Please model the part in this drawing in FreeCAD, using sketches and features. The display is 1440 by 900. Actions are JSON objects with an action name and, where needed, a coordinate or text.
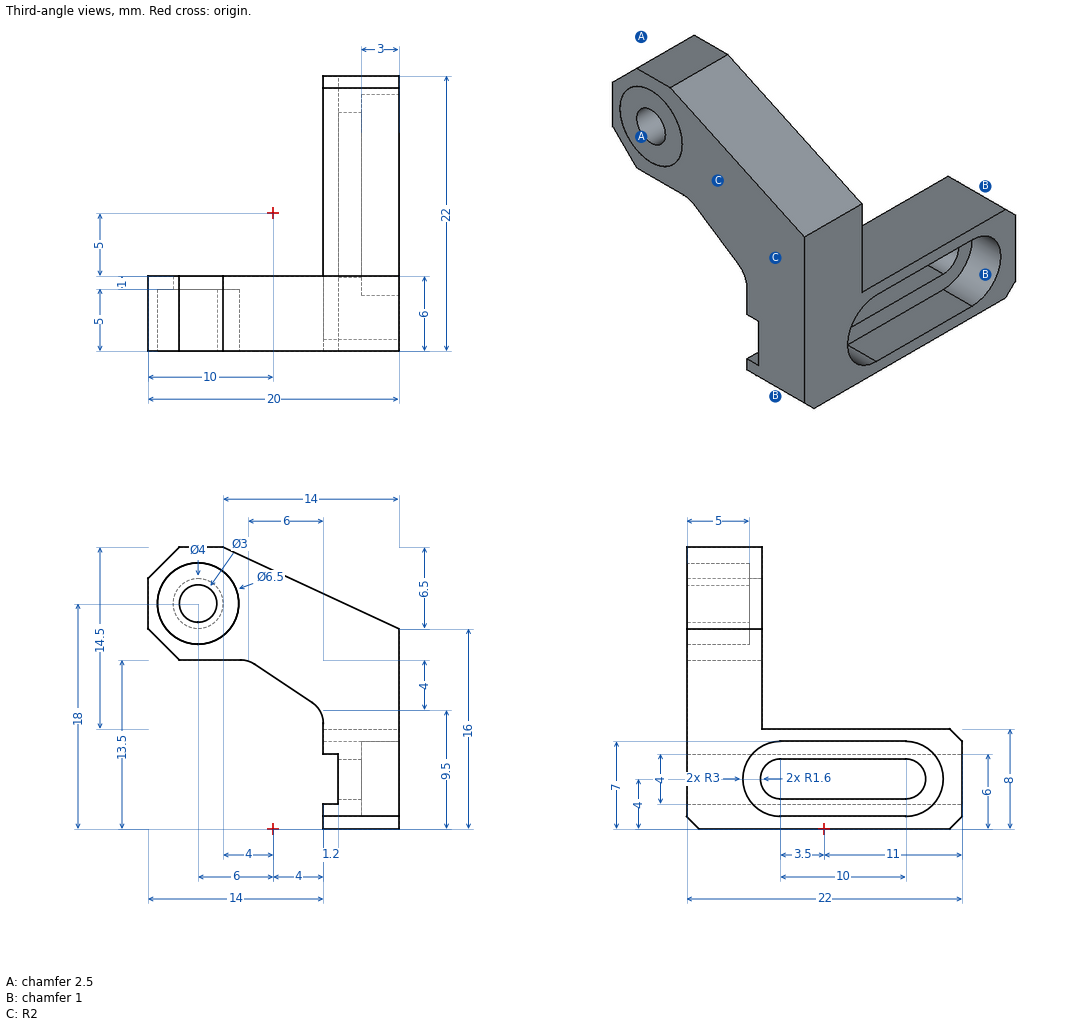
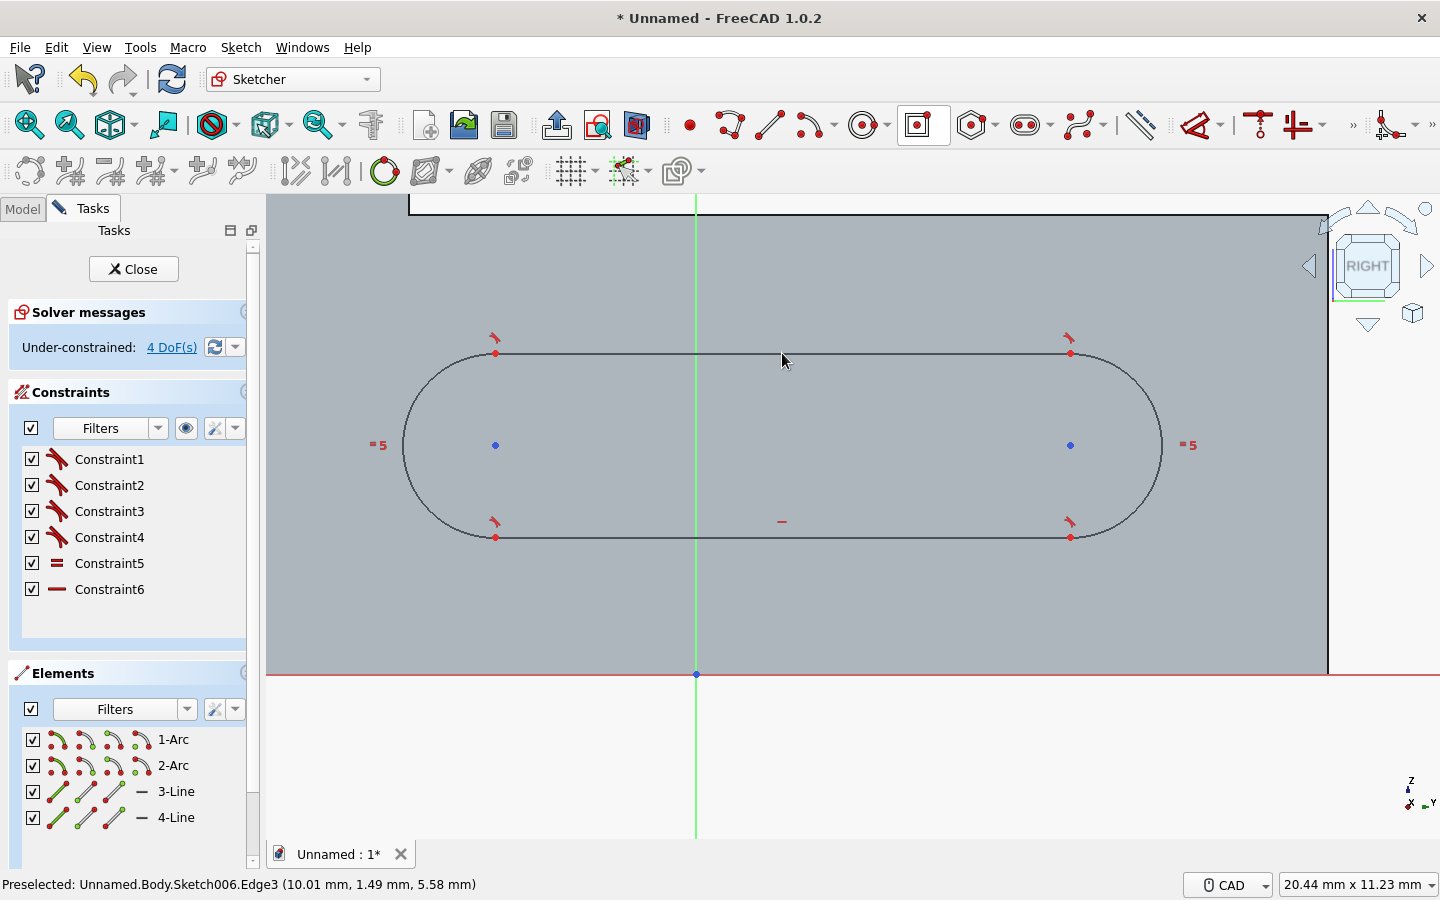
{"action": "left_click", "coordinate": [1196, 126]}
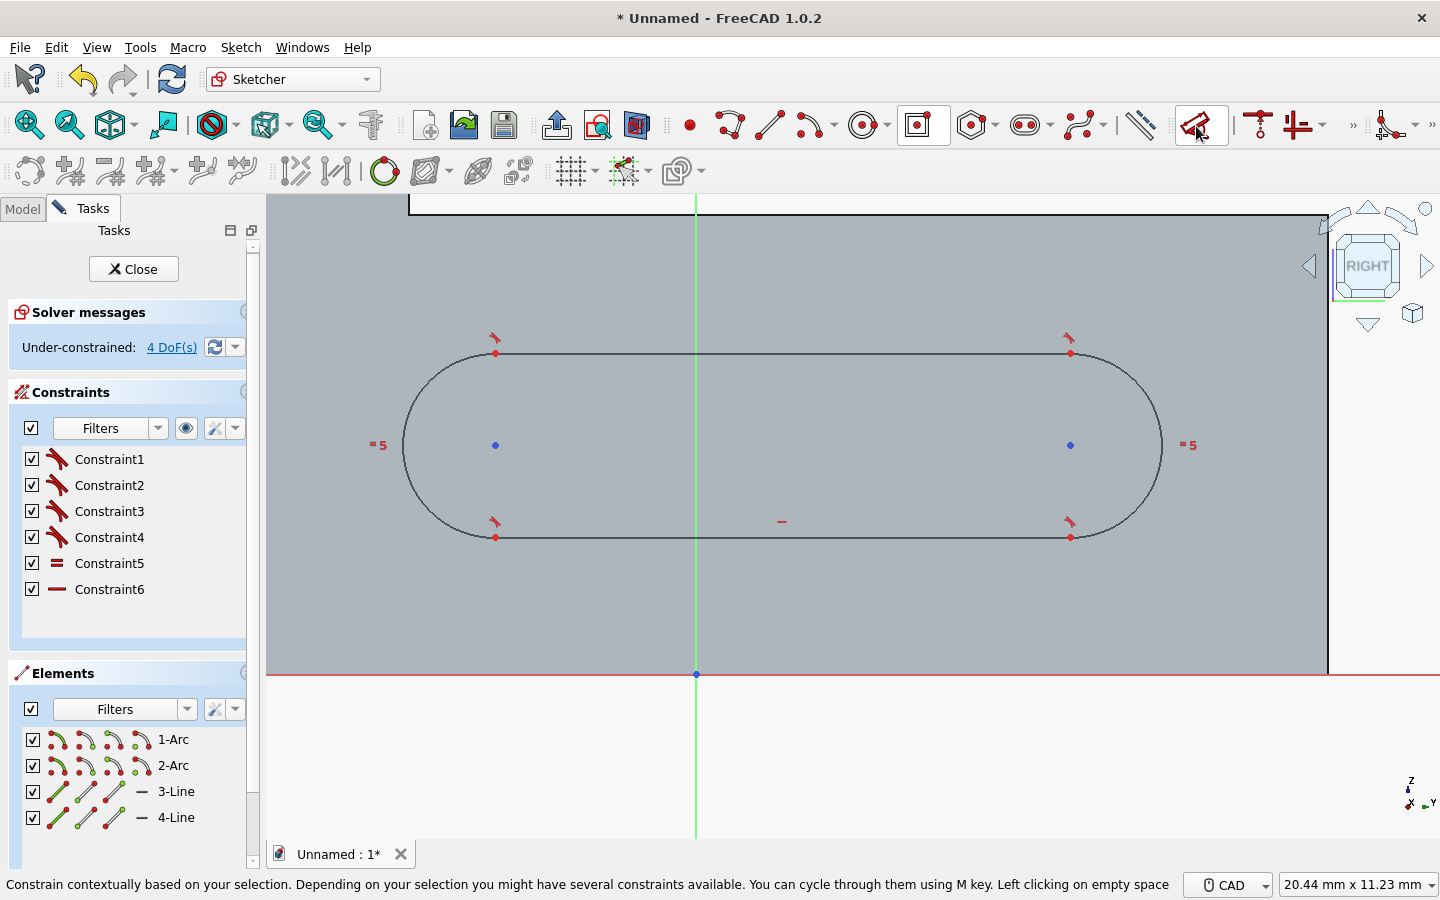
{"action": "left_click", "coordinate": [421, 392]}
{"action": "left_click", "coordinate": [395, 373]}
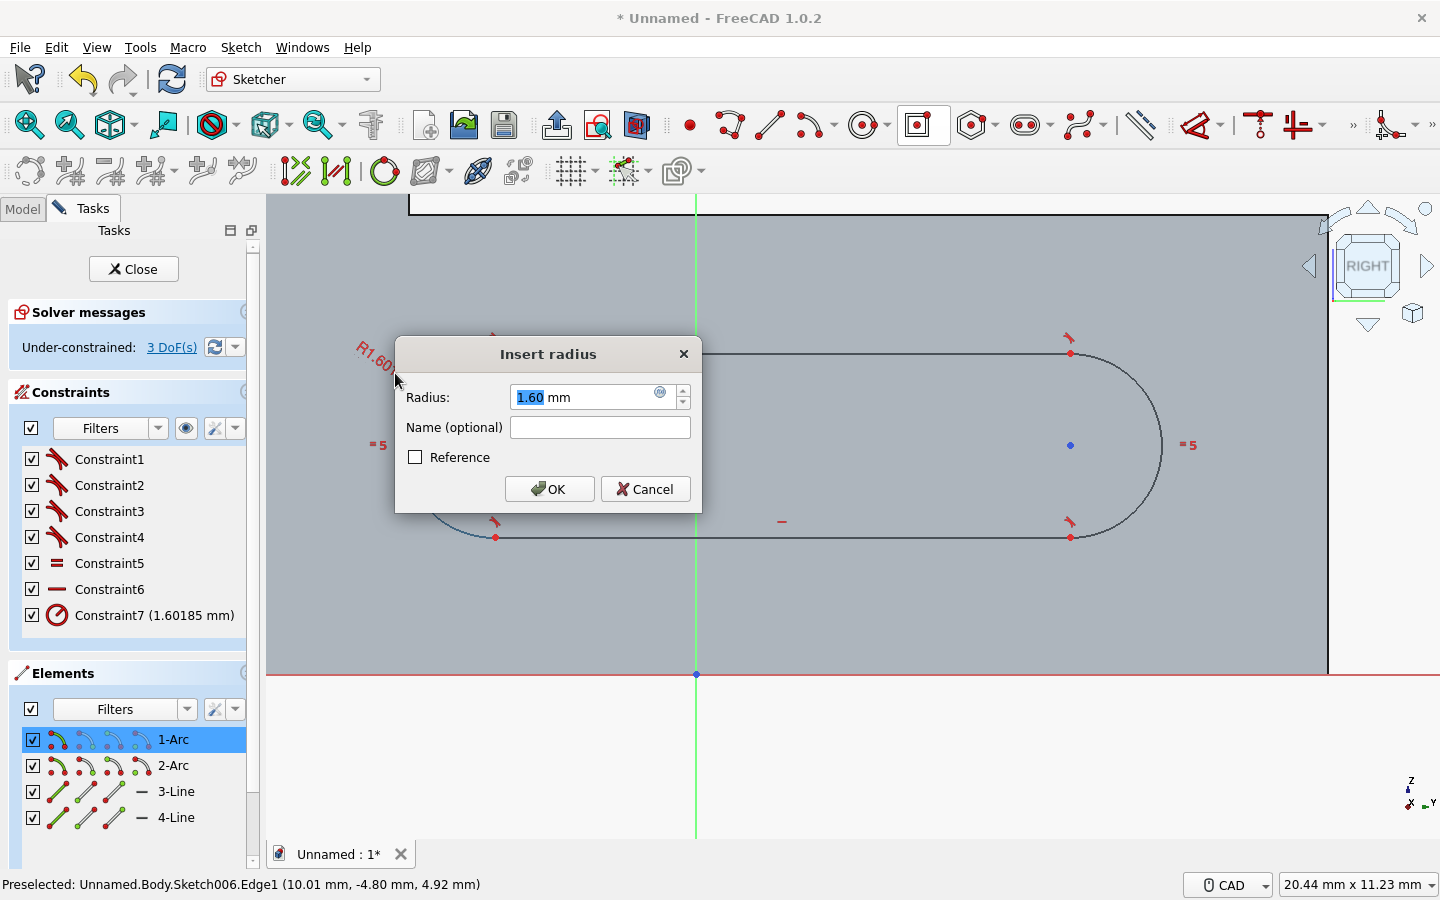
{"action": "type", "text": "1.6"}
{"action": "key", "text": "Return"}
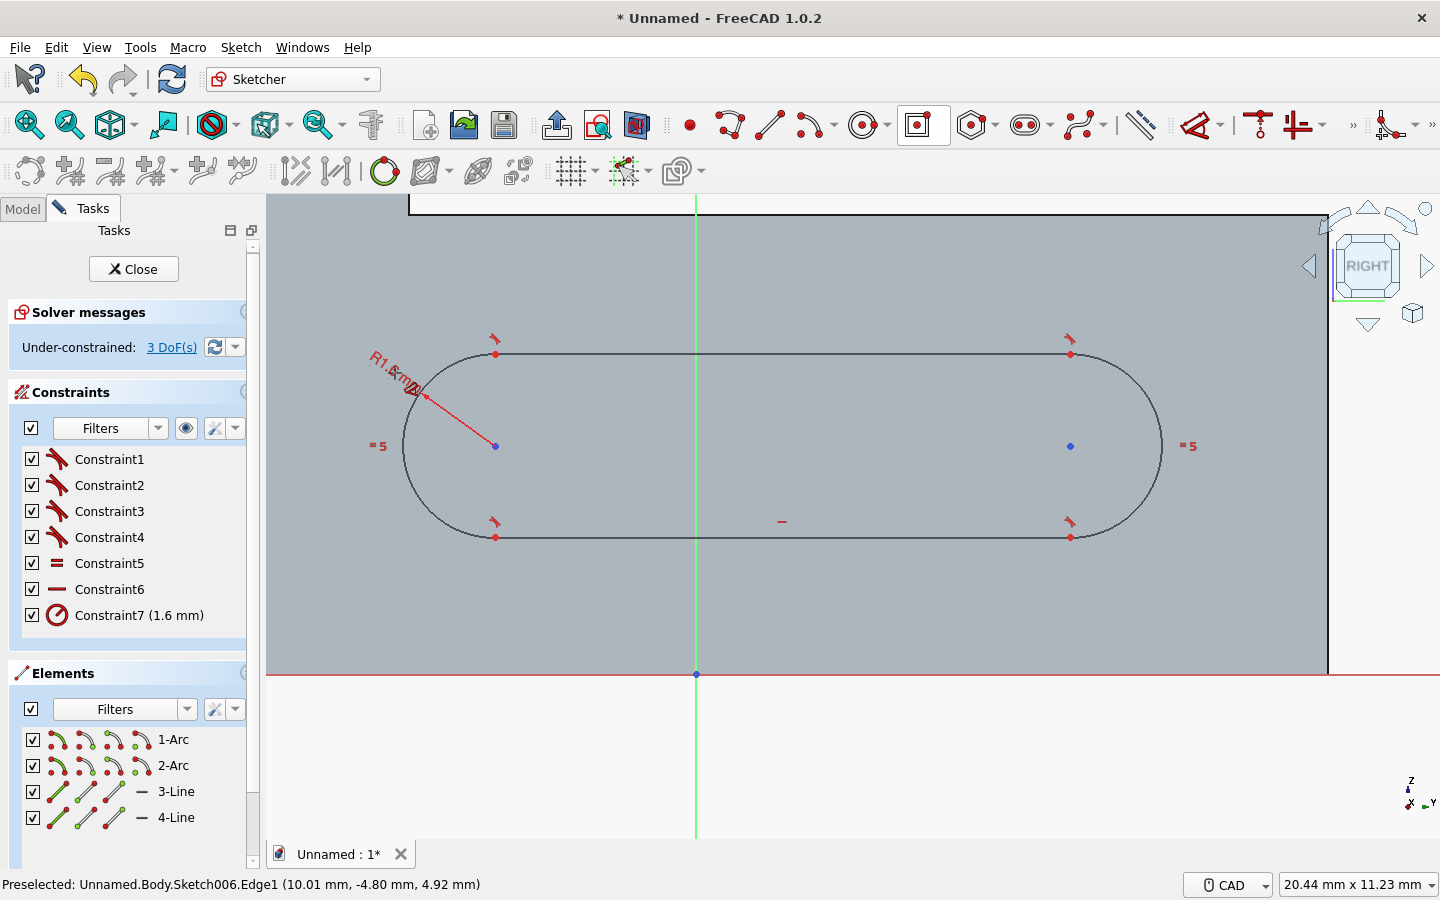
{"action": "left_click", "coordinate": [668, 354]}
{"action": "left_click", "coordinate": [783, 320]}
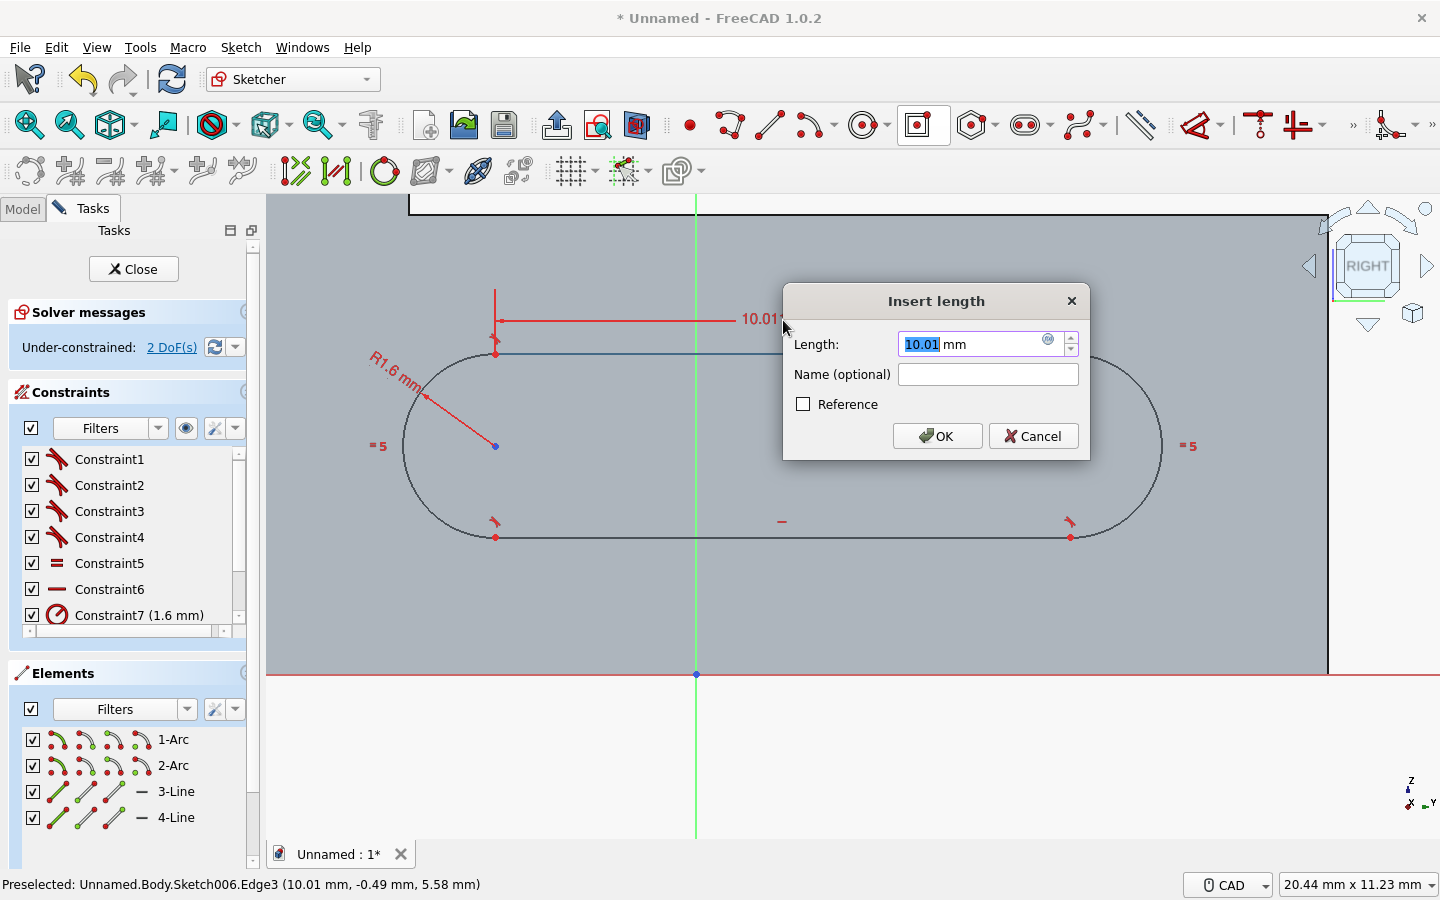
{"action": "type", "text": "10"}
{"action": "key", "text": "Return"}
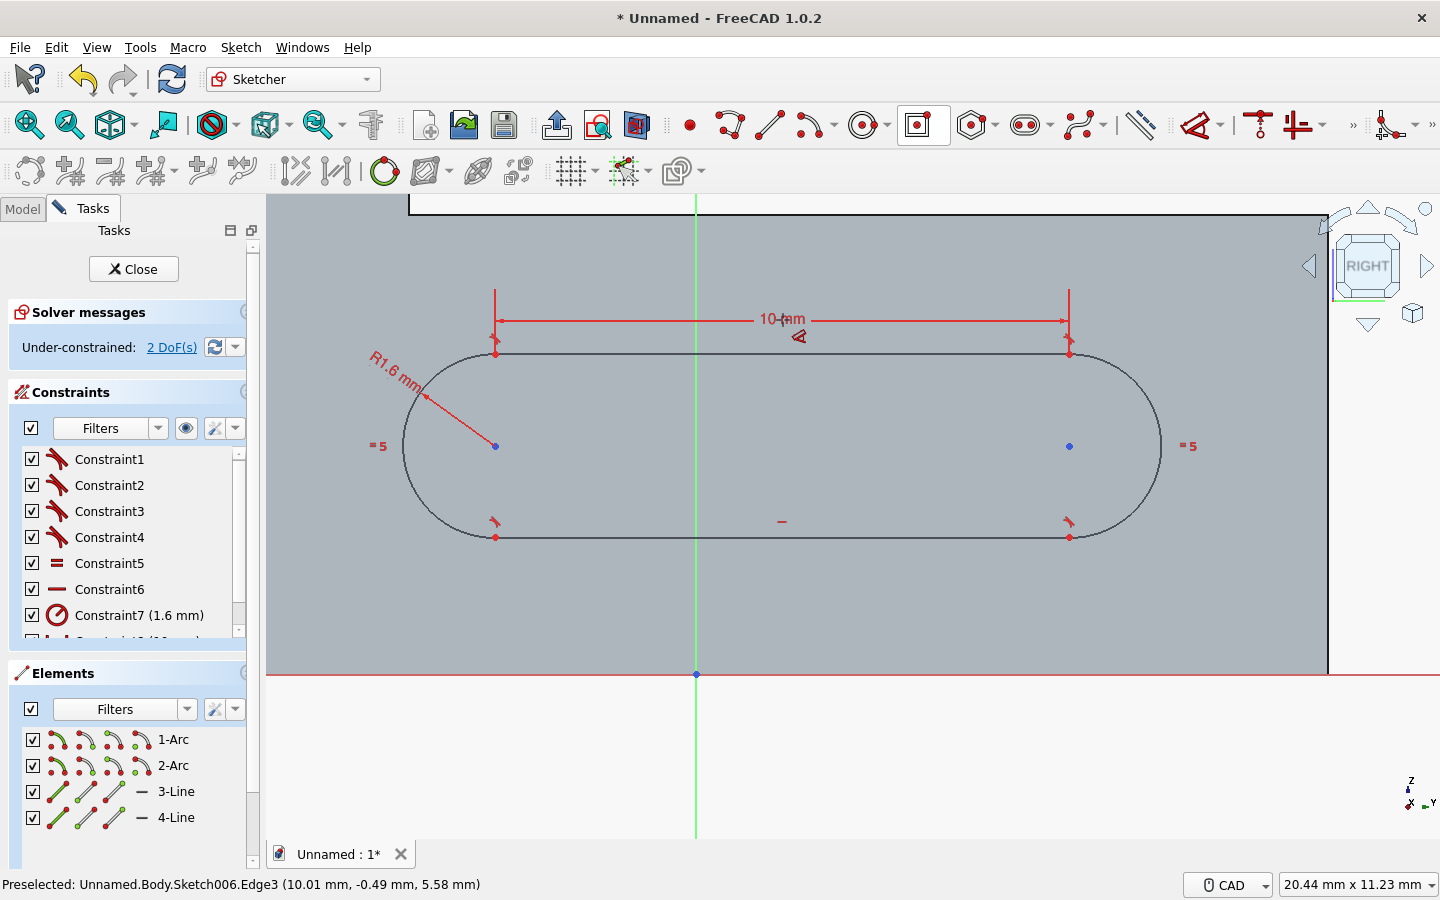
{"action": "left_click", "coordinate": [495, 446]}
{"action": "left_click", "coordinate": [461, 560]}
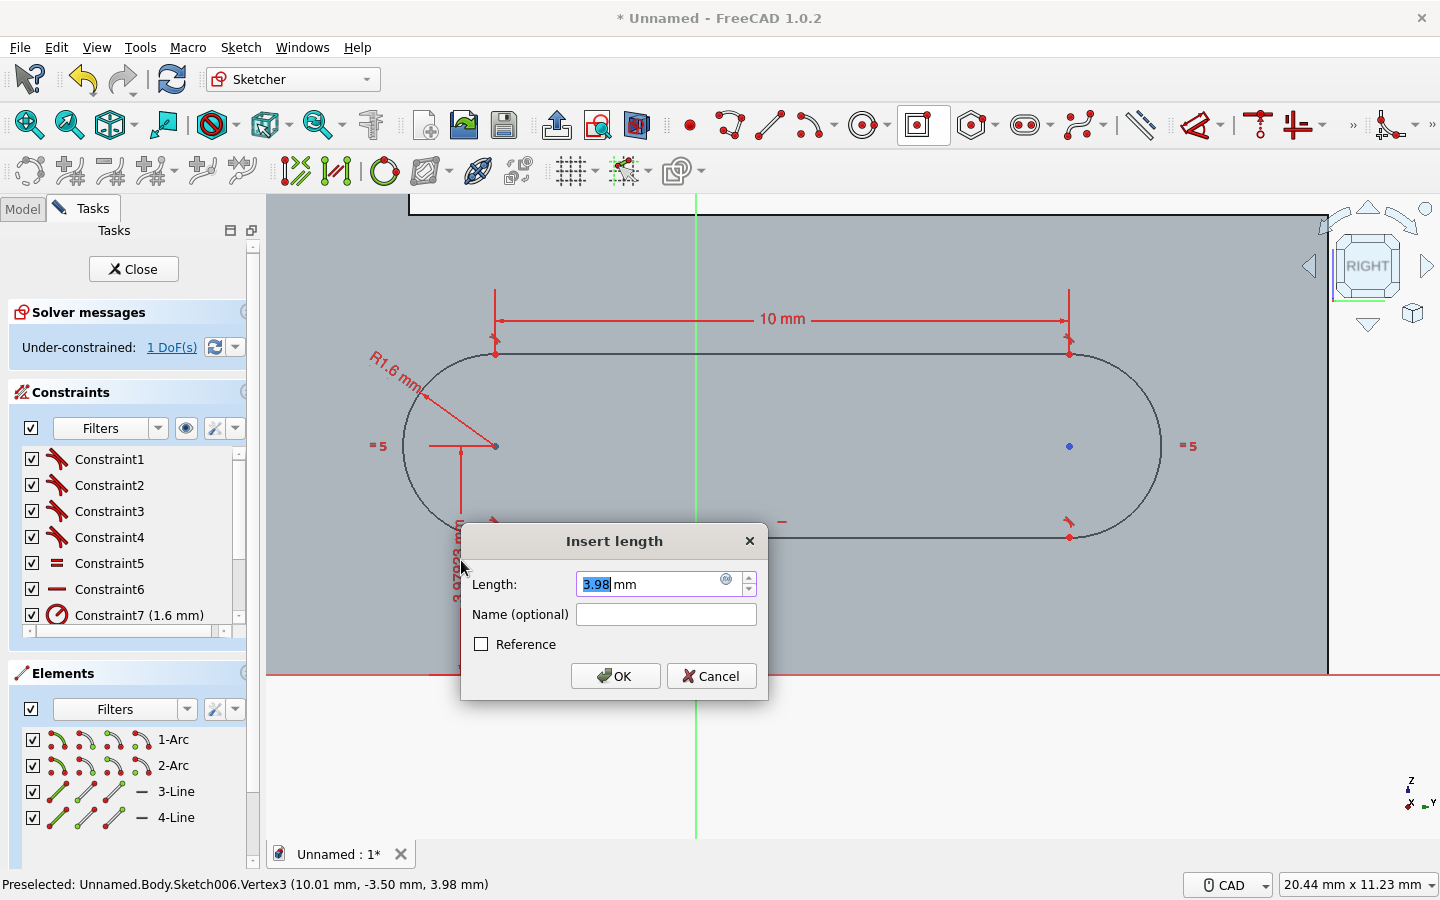
{"action": "type", "text": "4"}
{"action": "key", "text": "Return"}